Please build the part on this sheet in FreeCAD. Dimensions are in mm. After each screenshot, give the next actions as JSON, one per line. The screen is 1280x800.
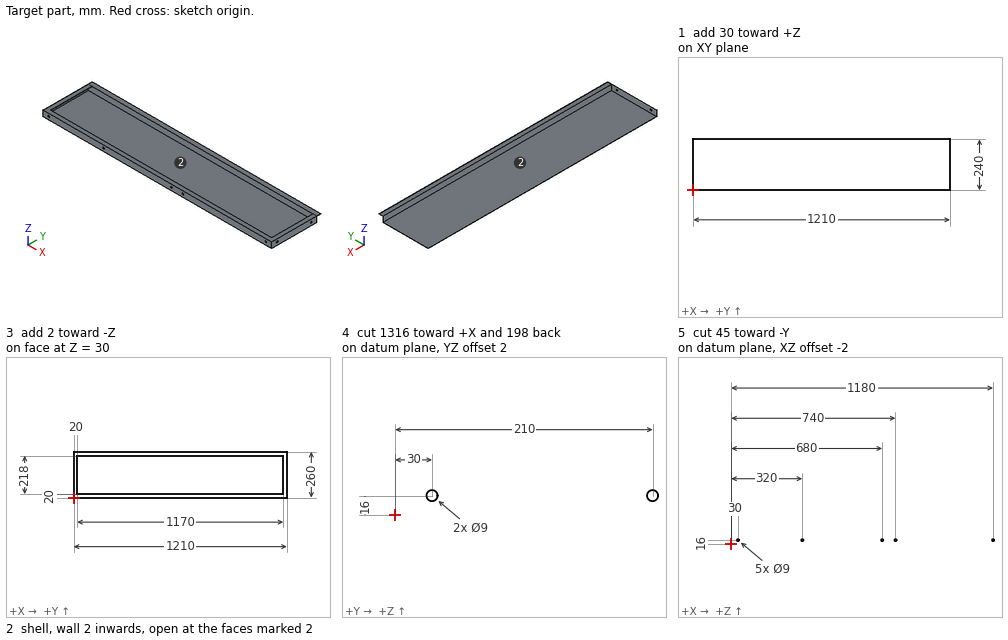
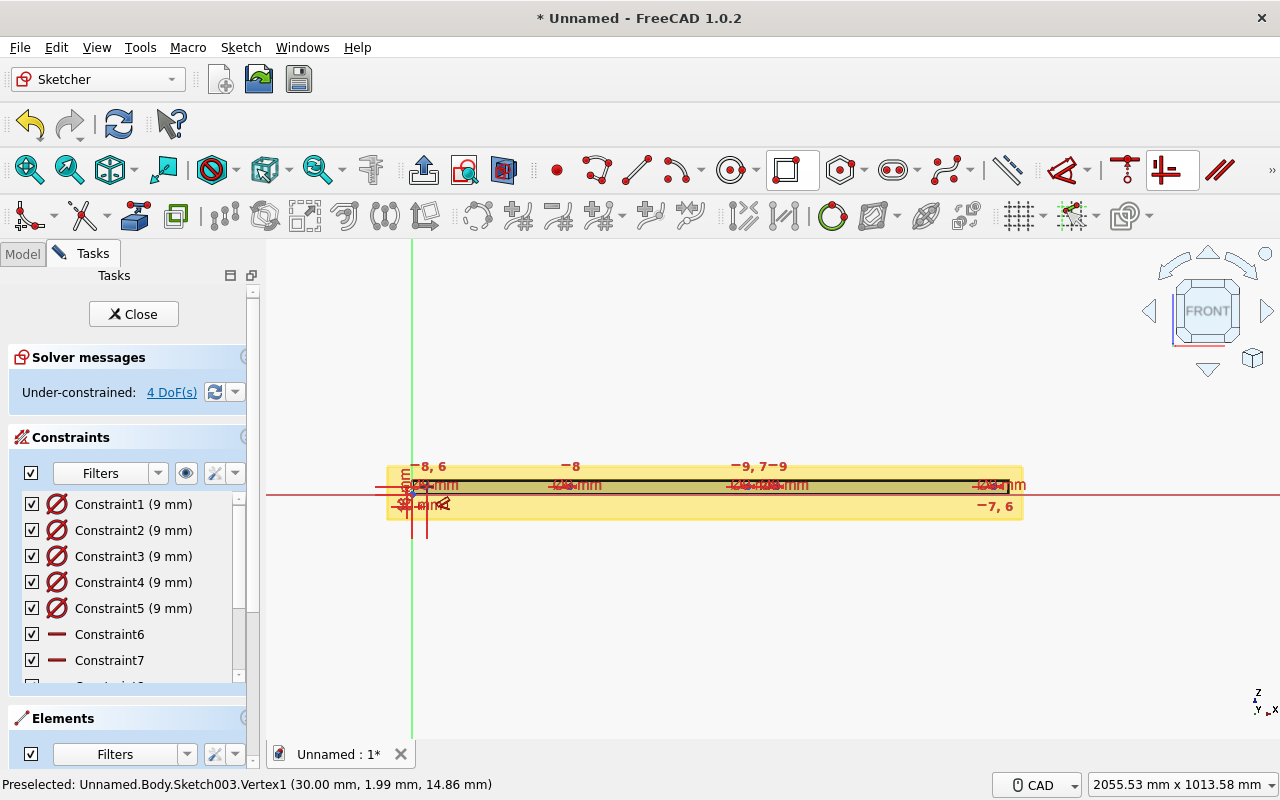
{"action": "left_click", "coordinate": [748, 487]}
{"action": "left_click", "coordinate": [580, 529]}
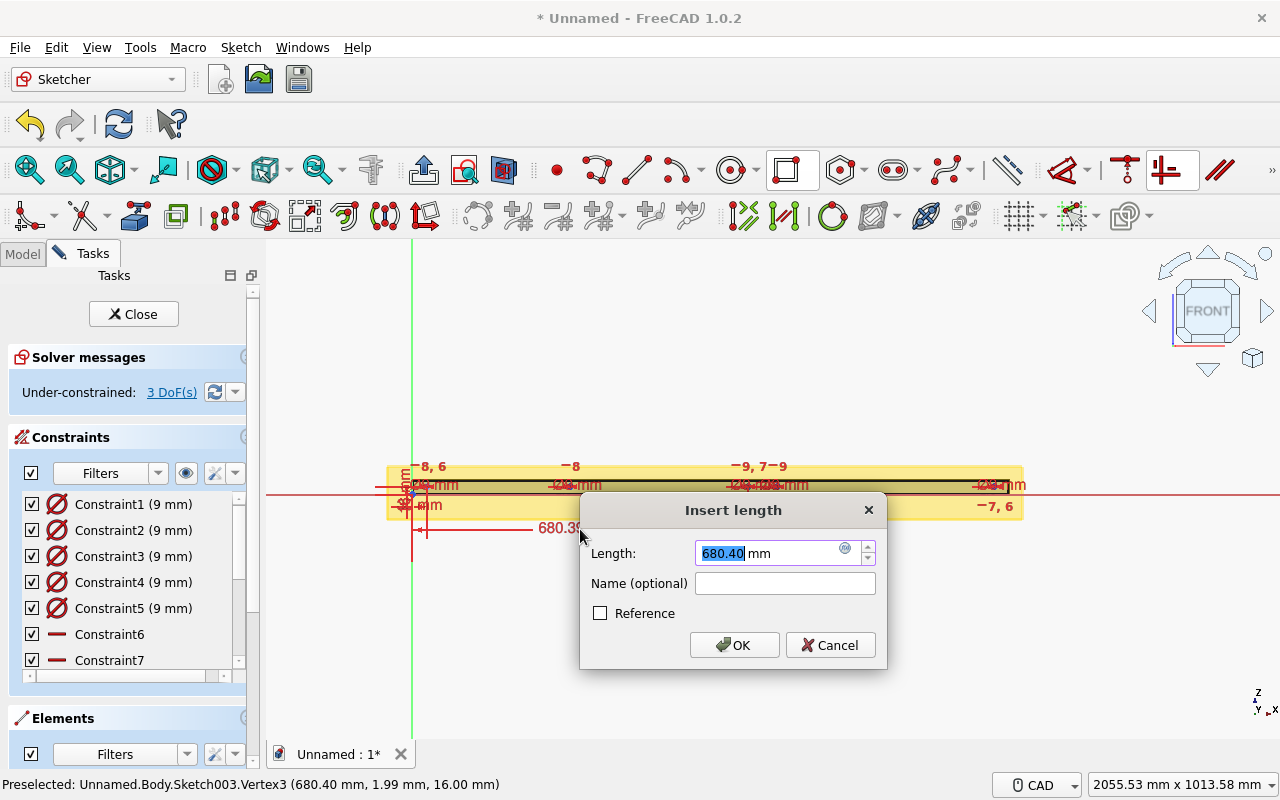
{"action": "type", "text": "680"}
{"action": "key", "text": "Return"}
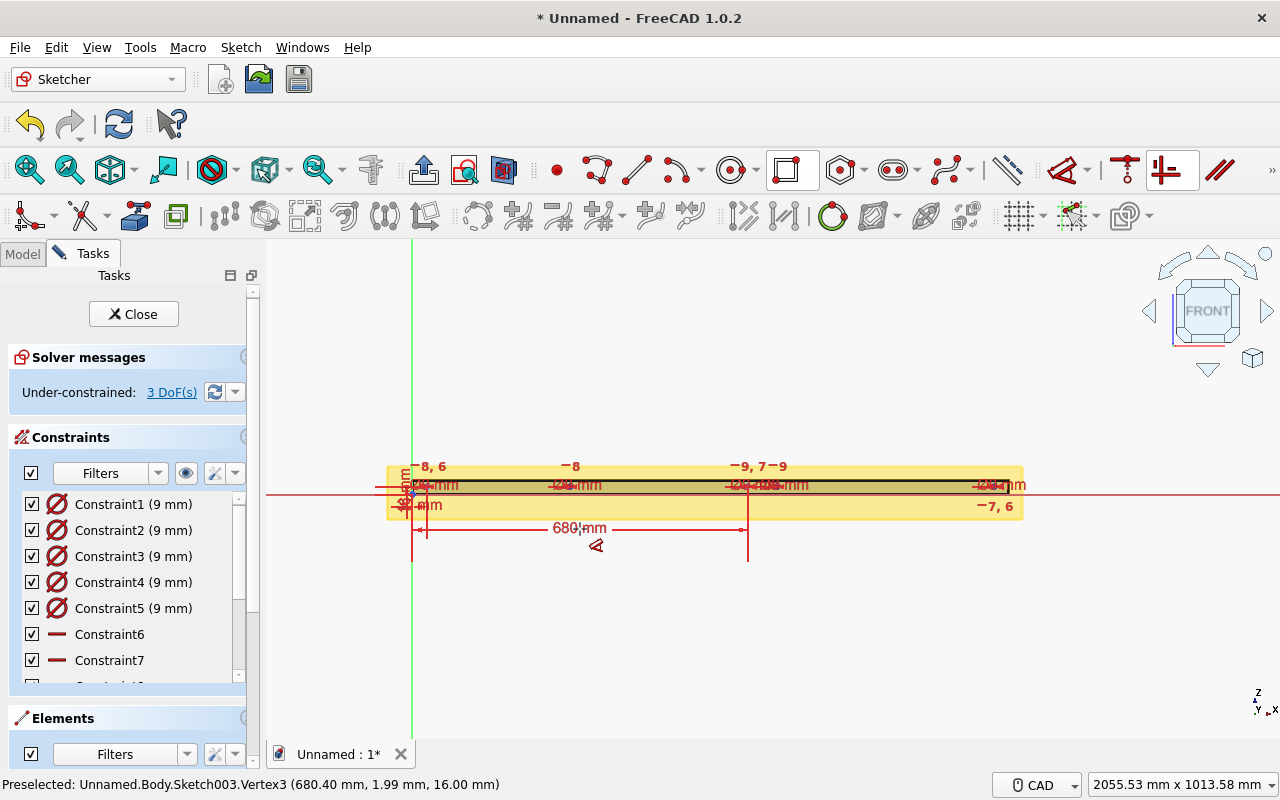
{"action": "left_click", "coordinate": [570, 487]}
{"action": "left_click", "coordinate": [491, 529]}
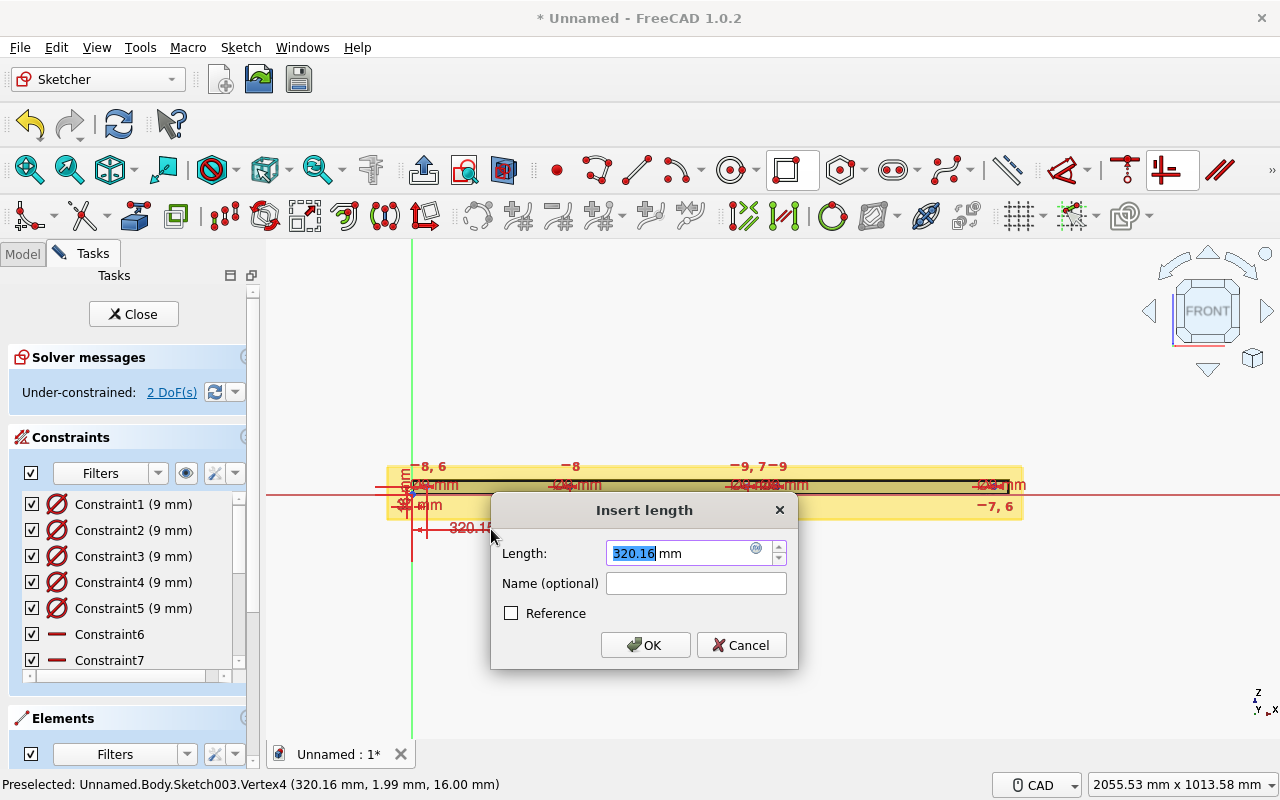
{"action": "type", "text": "320"}
{"action": "key", "text": "Return"}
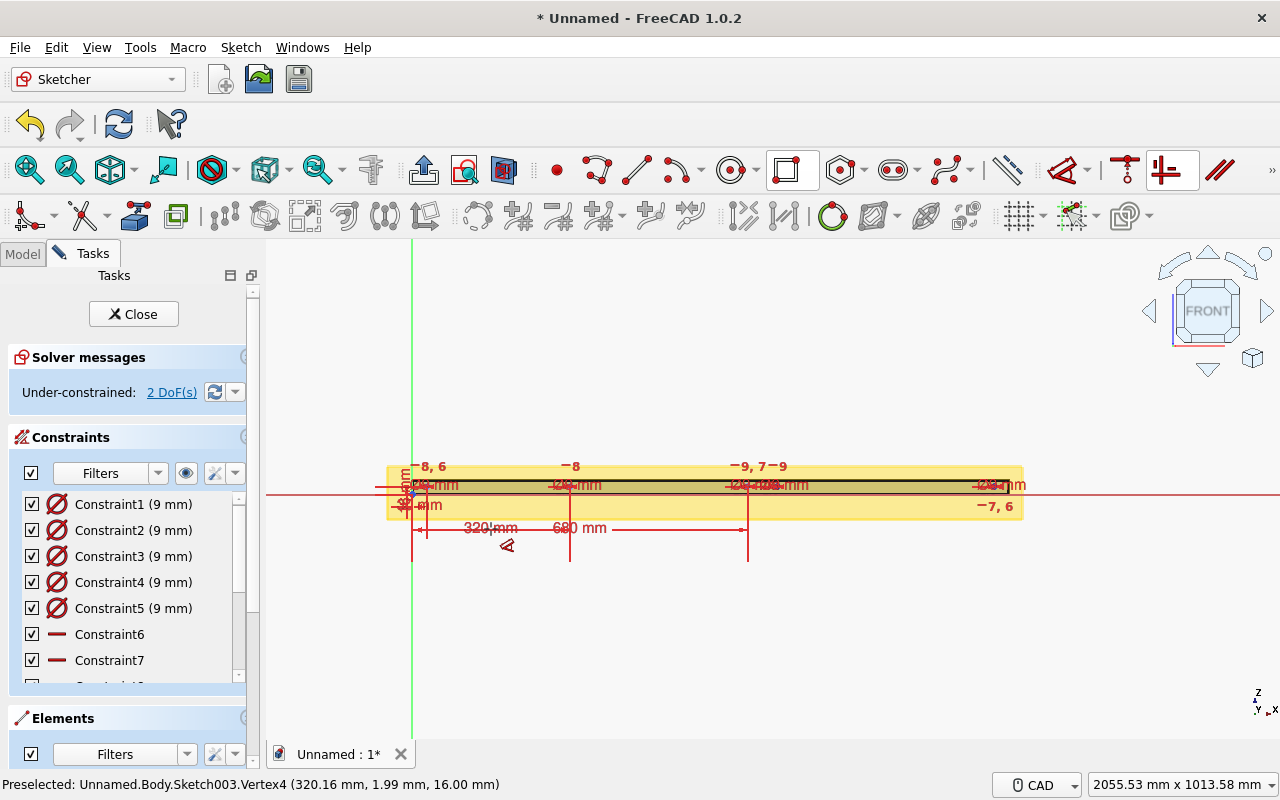
{"action": "left_click", "coordinate": [777, 487]}
{"action": "left_click", "coordinate": [679, 529]}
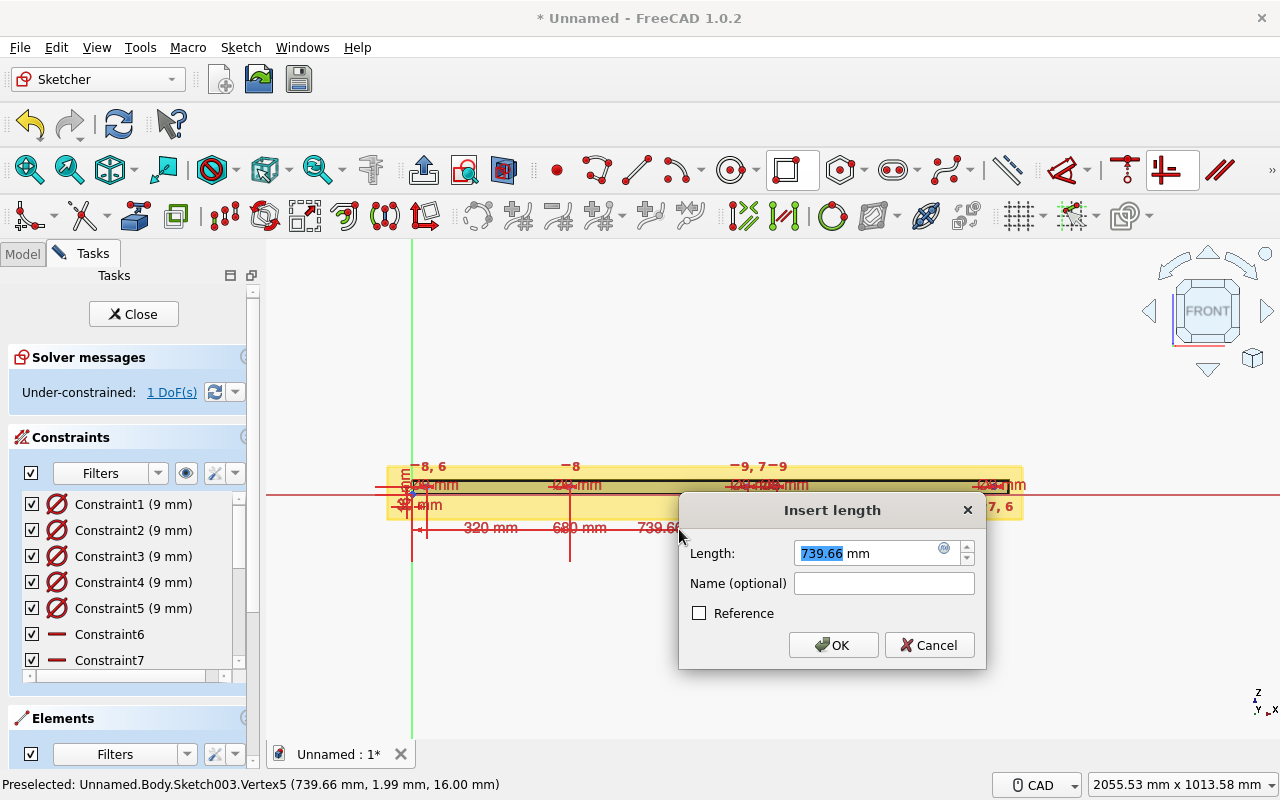
{"action": "type", "text": "740"}
{"action": "key", "text": "Return"}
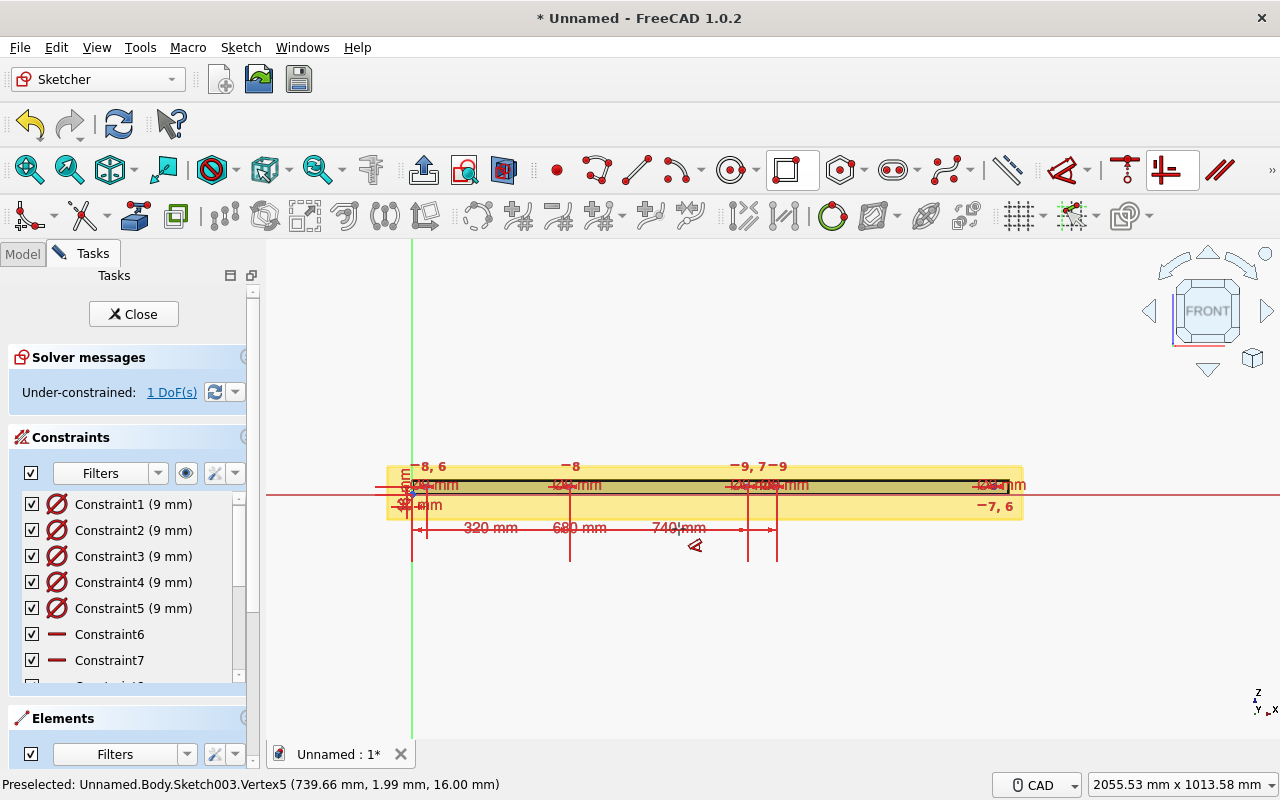
{"action": "left_click", "coordinate": [995, 487]}
{"action": "left_click", "coordinate": [837, 529]}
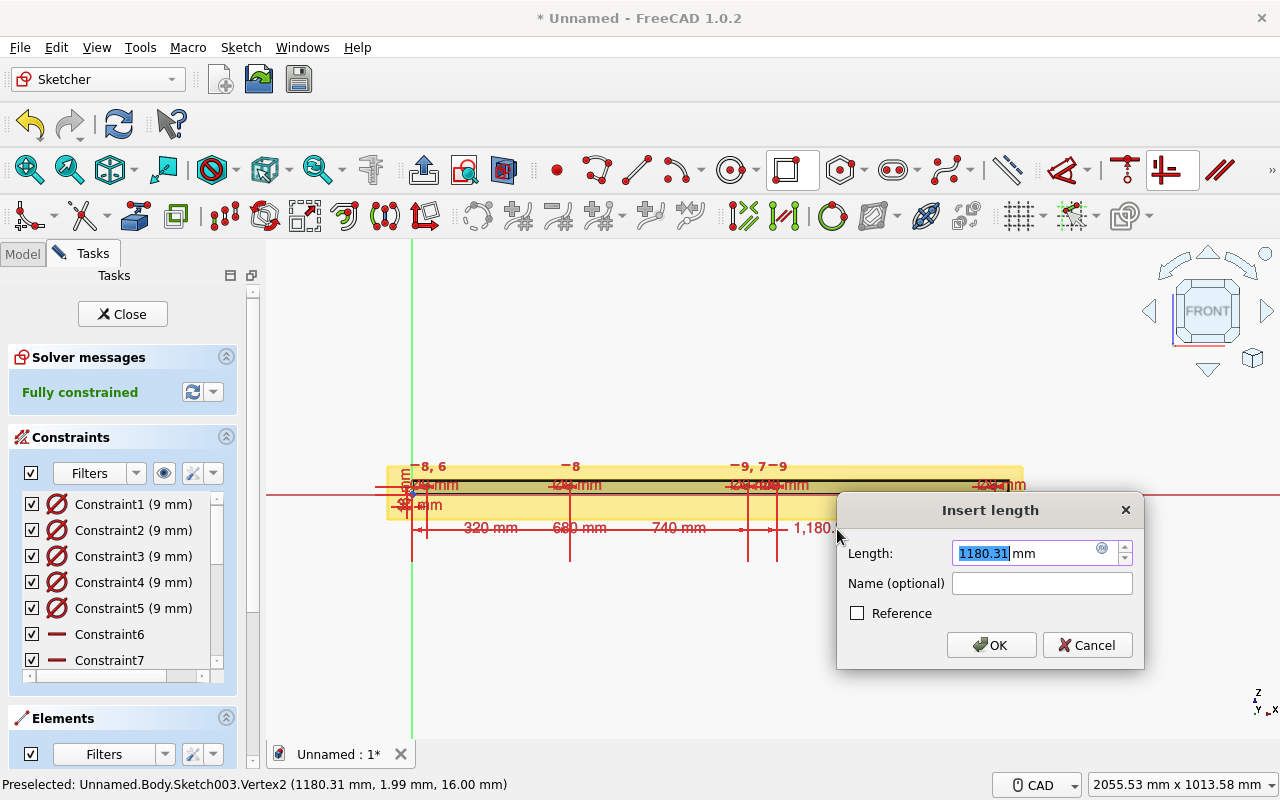
{"action": "type", "text": "1180"}
{"action": "key", "text": "Return"}
{"action": "key", "text": "Escape"}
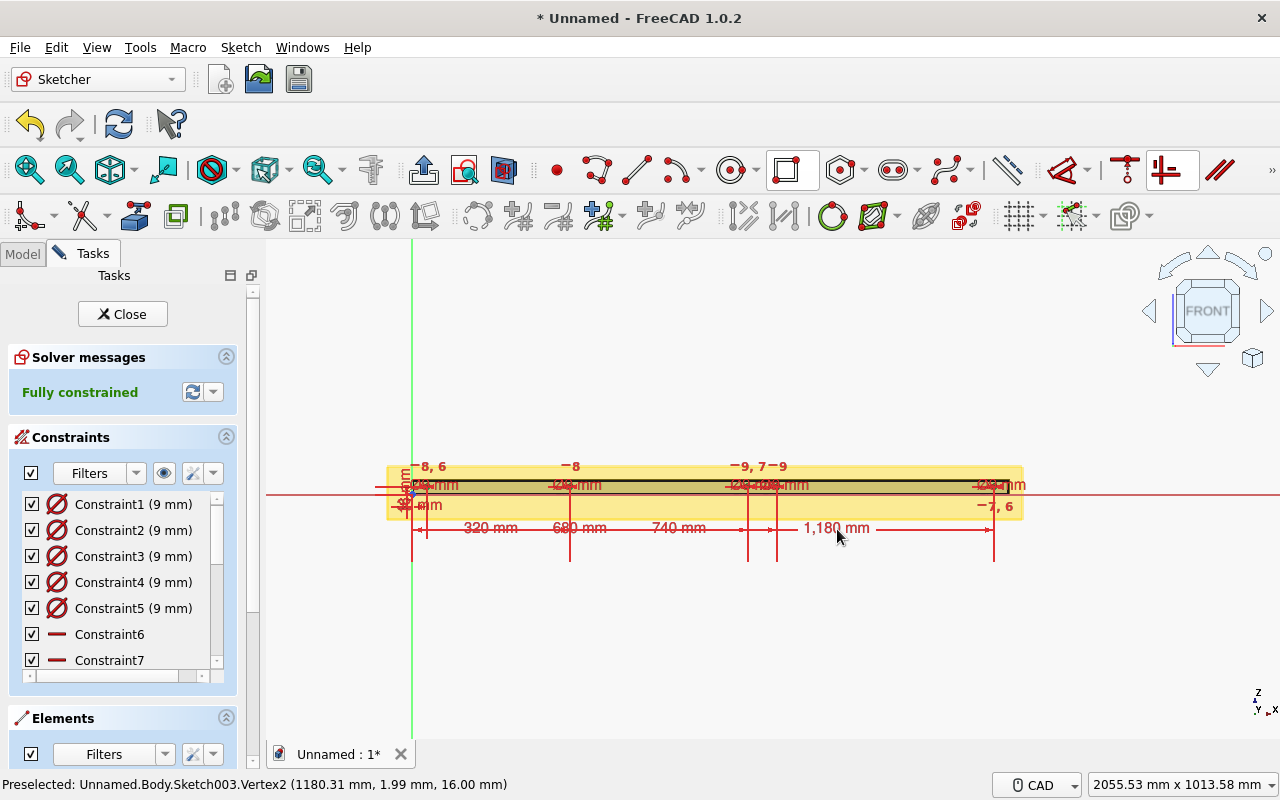
{"action": "left_click", "coordinate": [123, 314]}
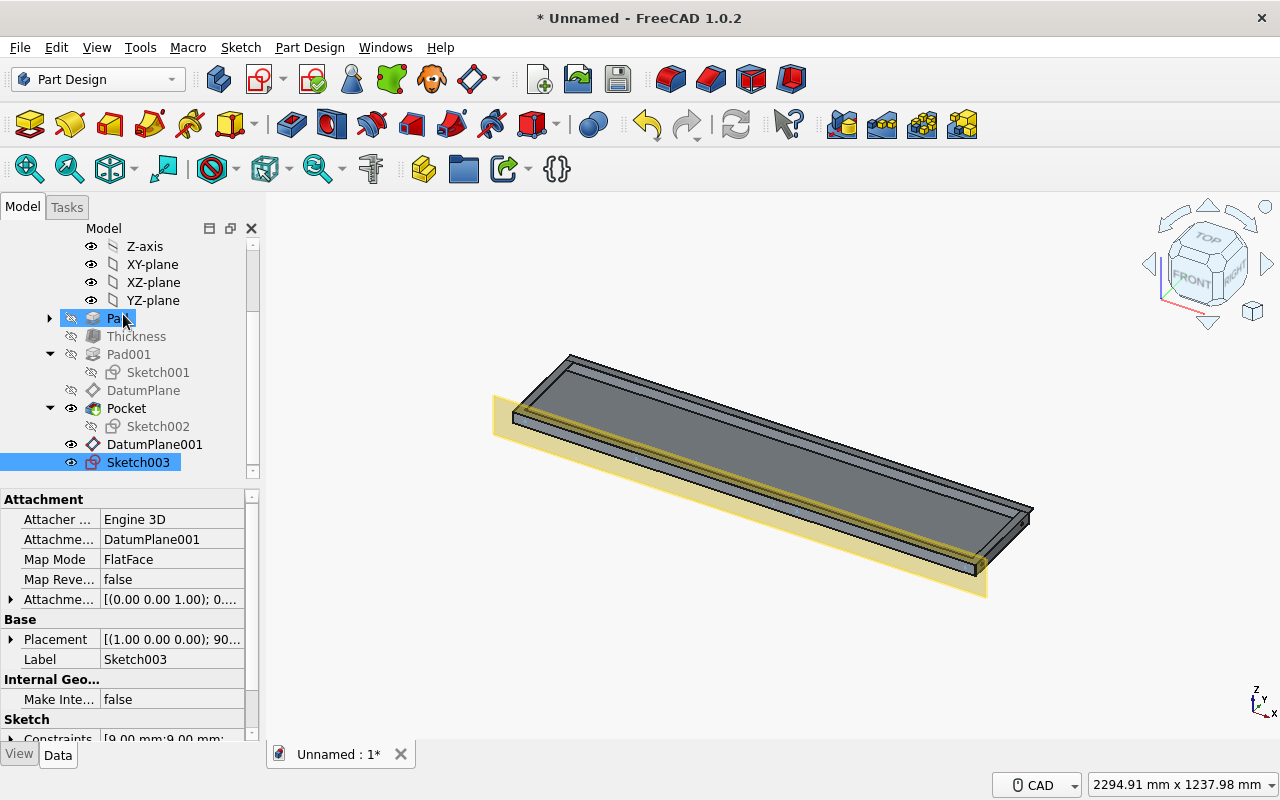
{"action": "left_click", "coordinate": [292, 124]}